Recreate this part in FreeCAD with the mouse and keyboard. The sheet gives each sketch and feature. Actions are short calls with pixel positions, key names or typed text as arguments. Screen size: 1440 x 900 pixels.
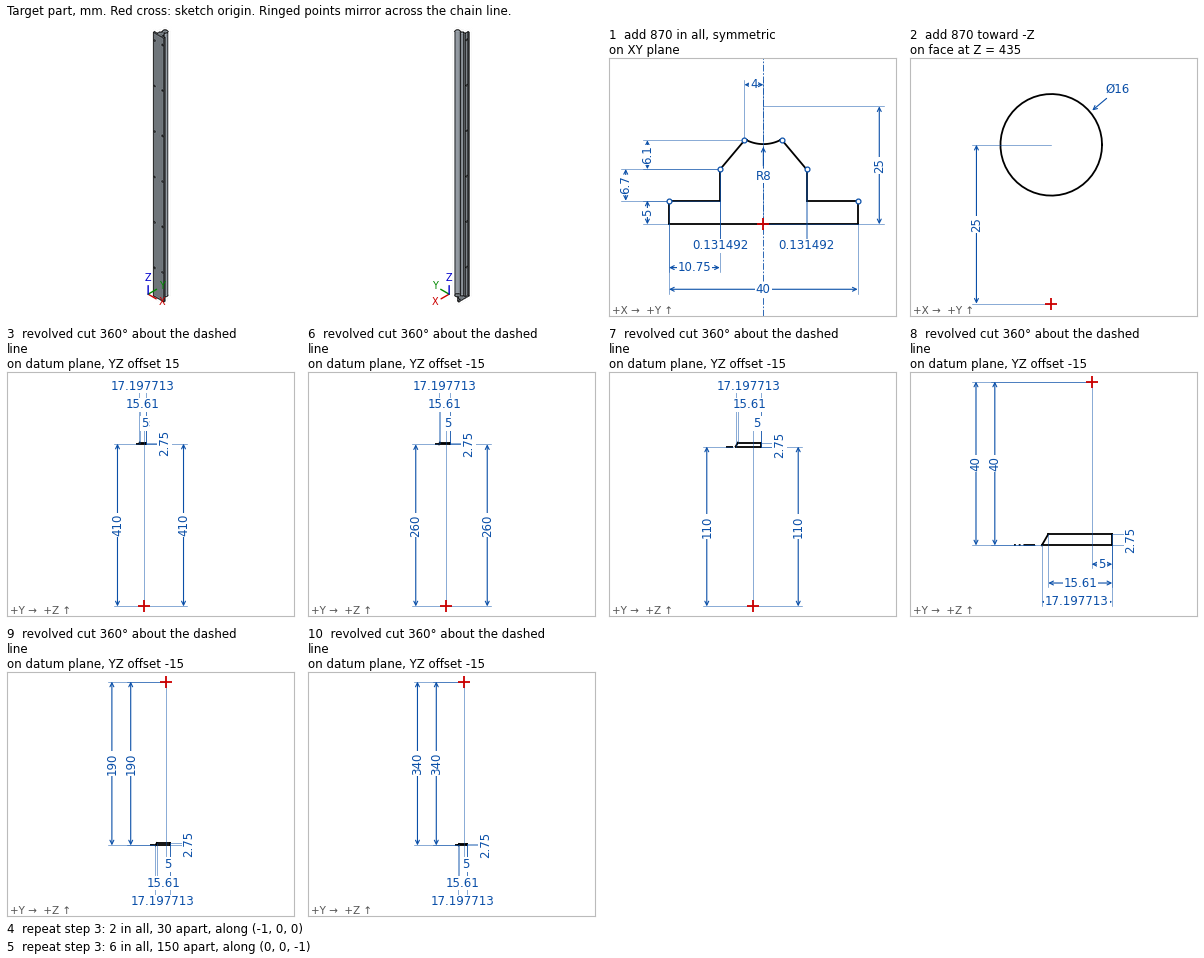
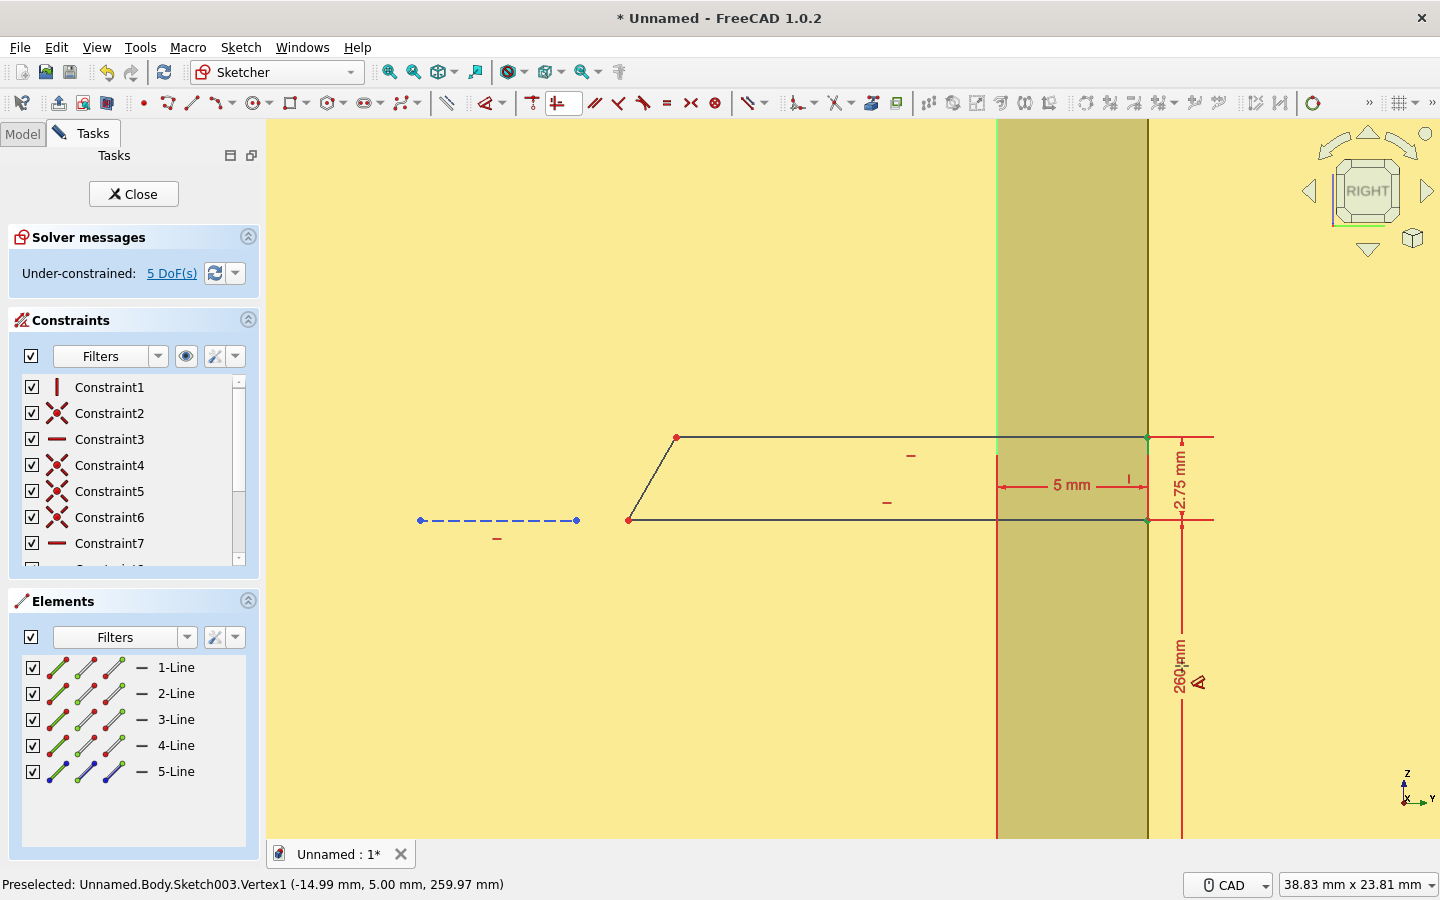
click(576, 521)
click(1031, 666)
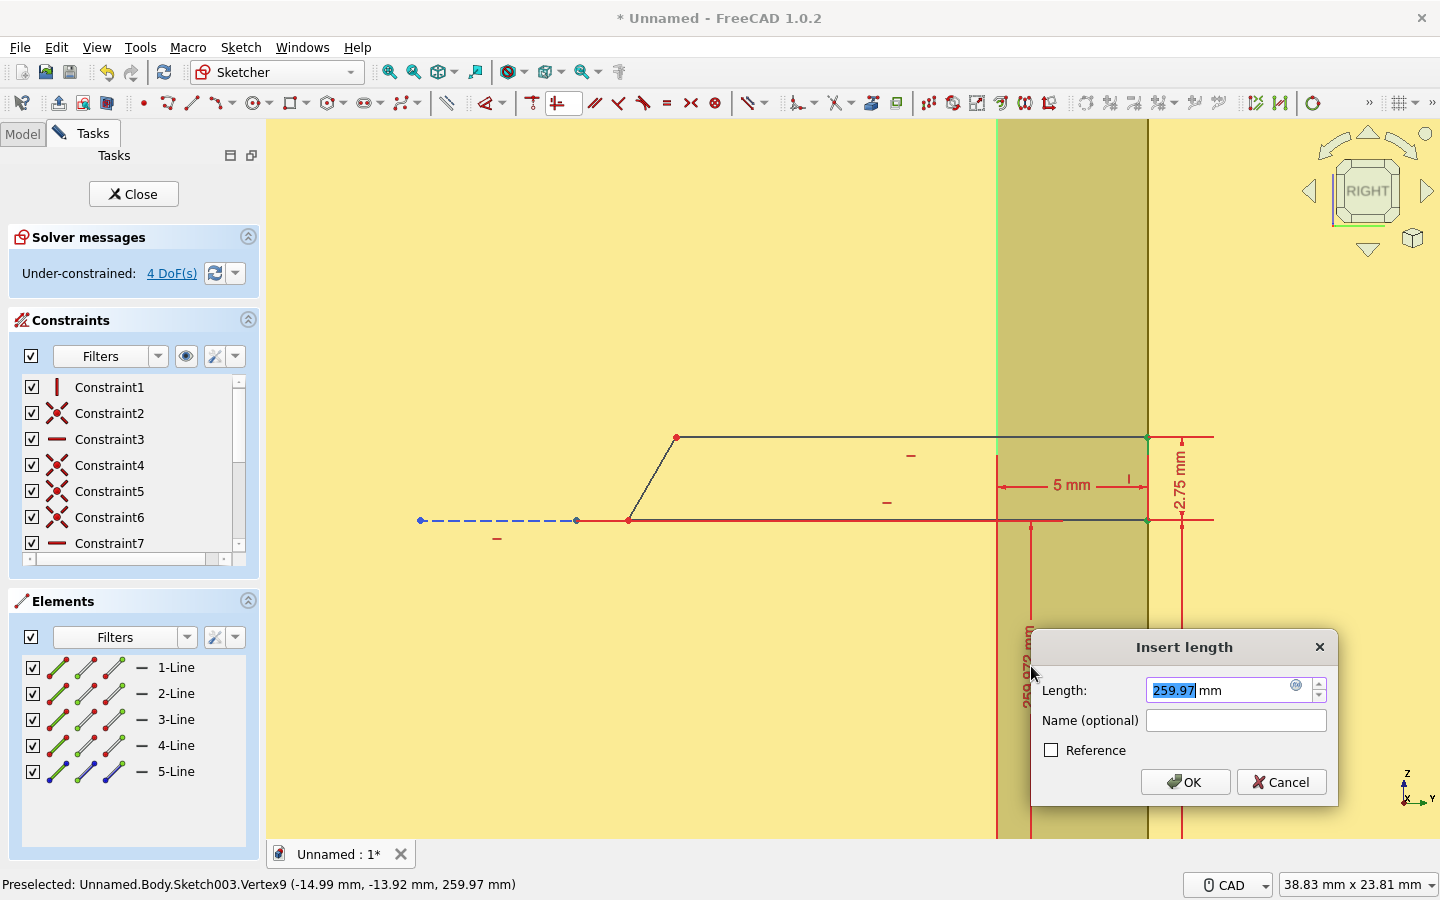
text(260)
key(Return)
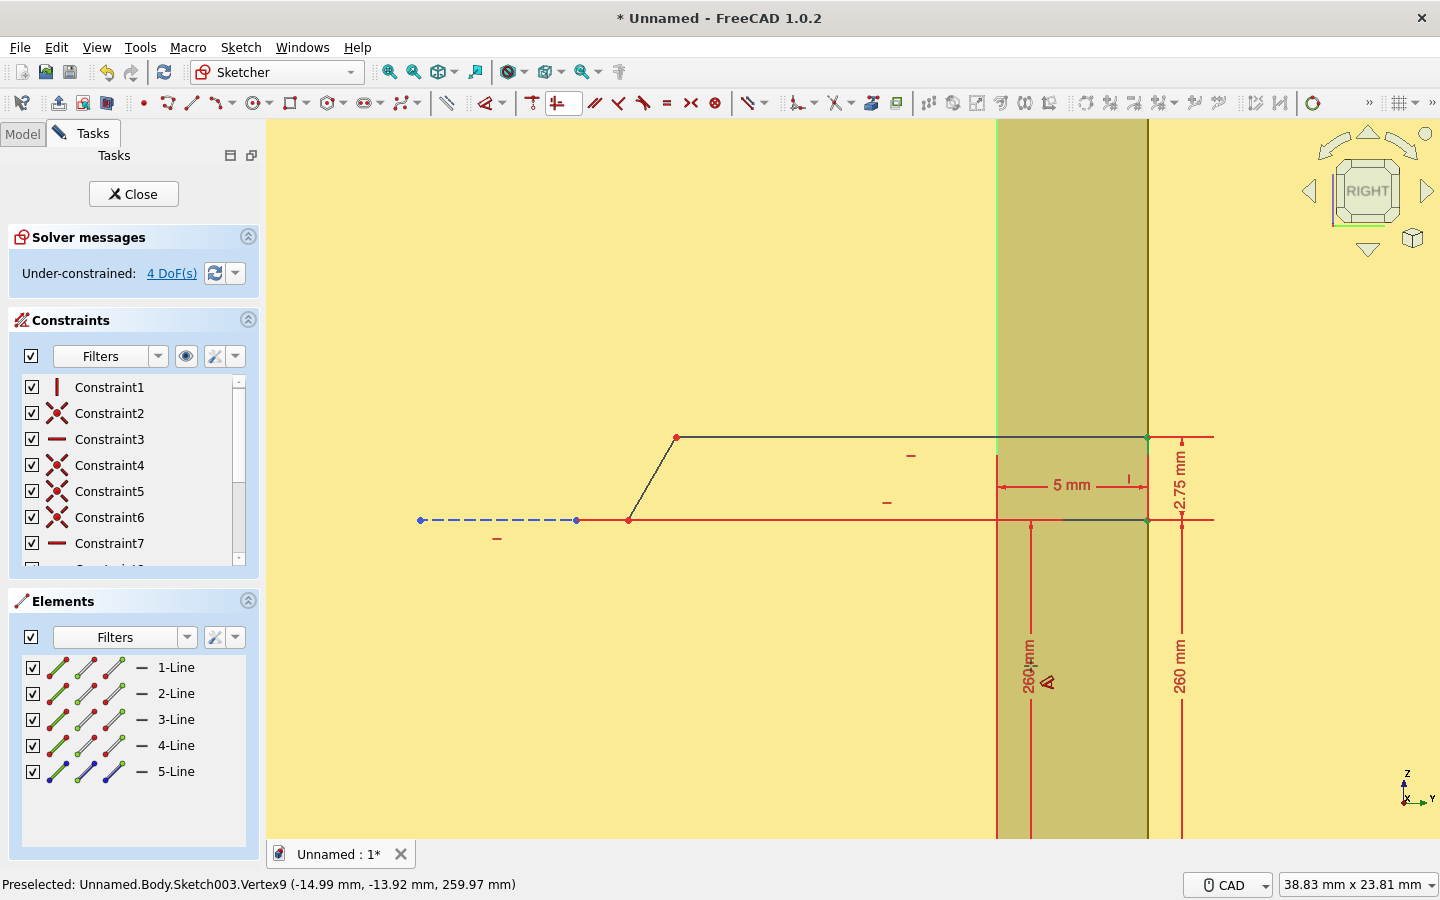
scroll(1006, 437, up, 2)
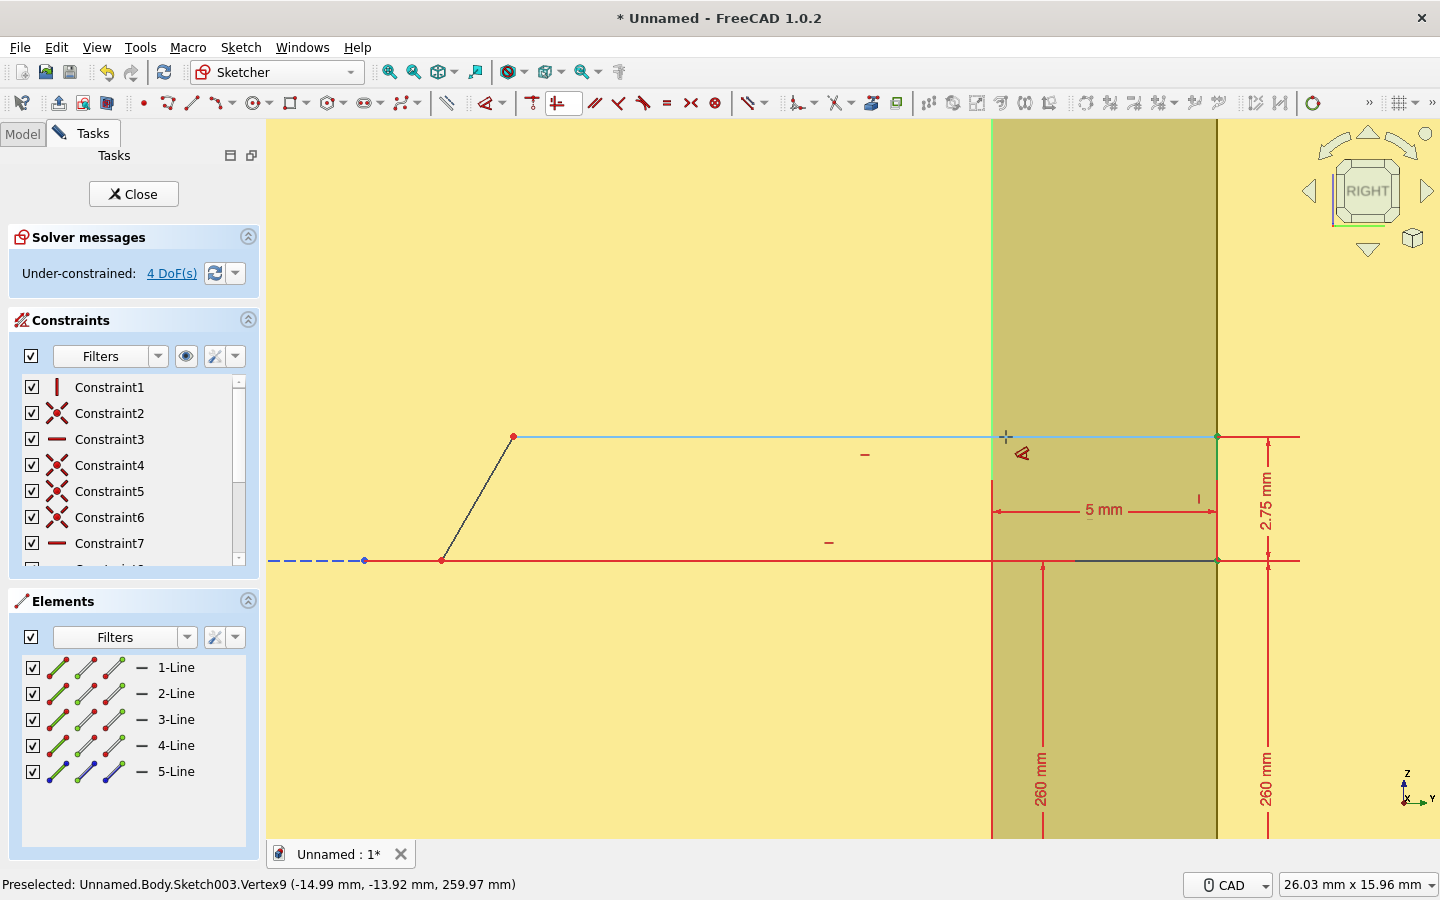
click(1006, 437)
click(865, 403)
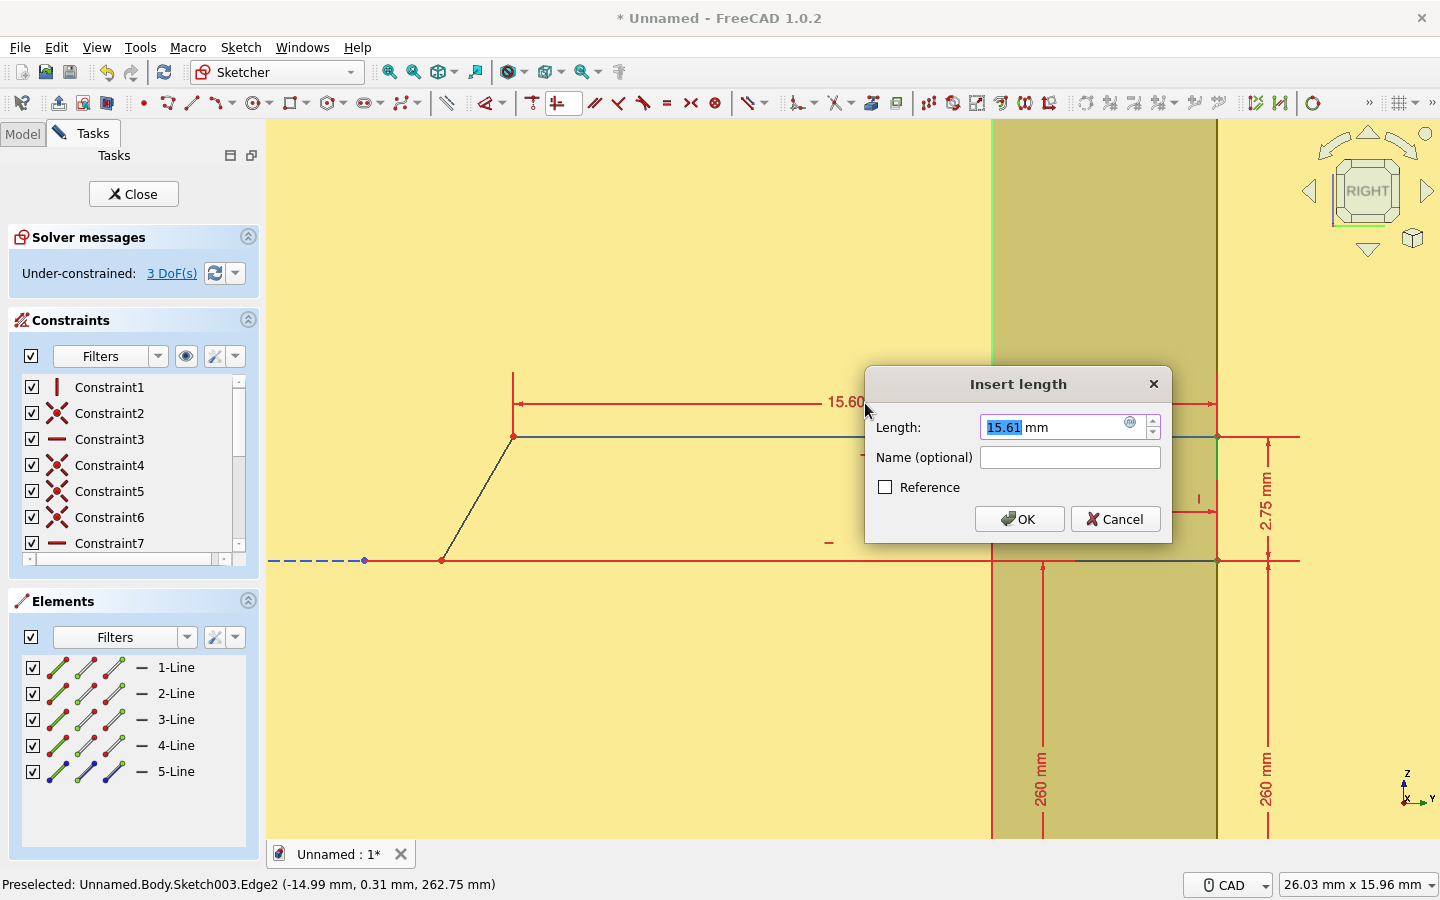
text(15.61)
key(Return)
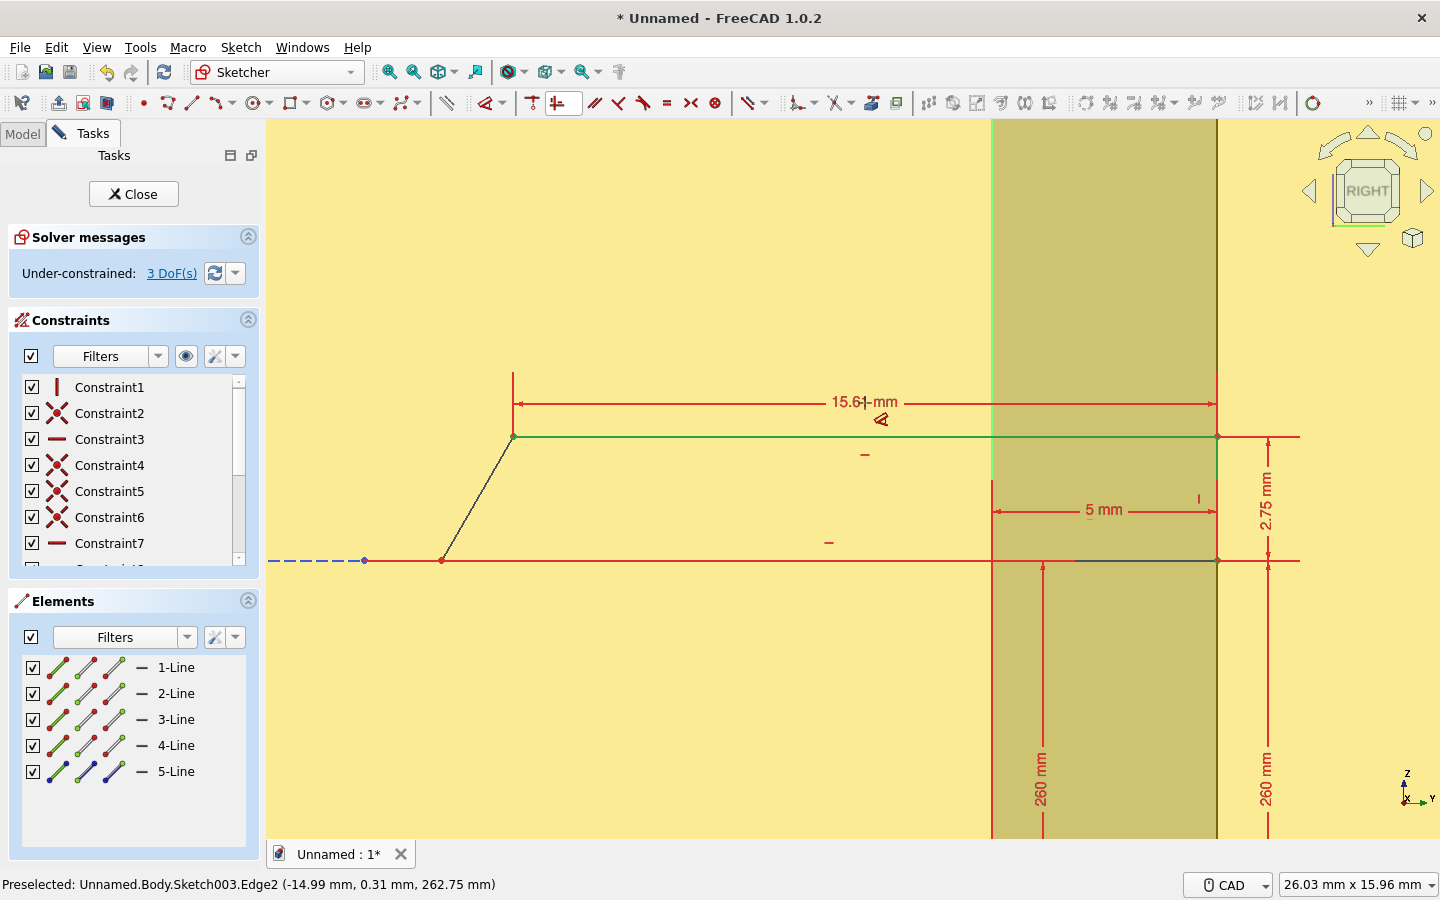
click(674, 561)
click(830, 595)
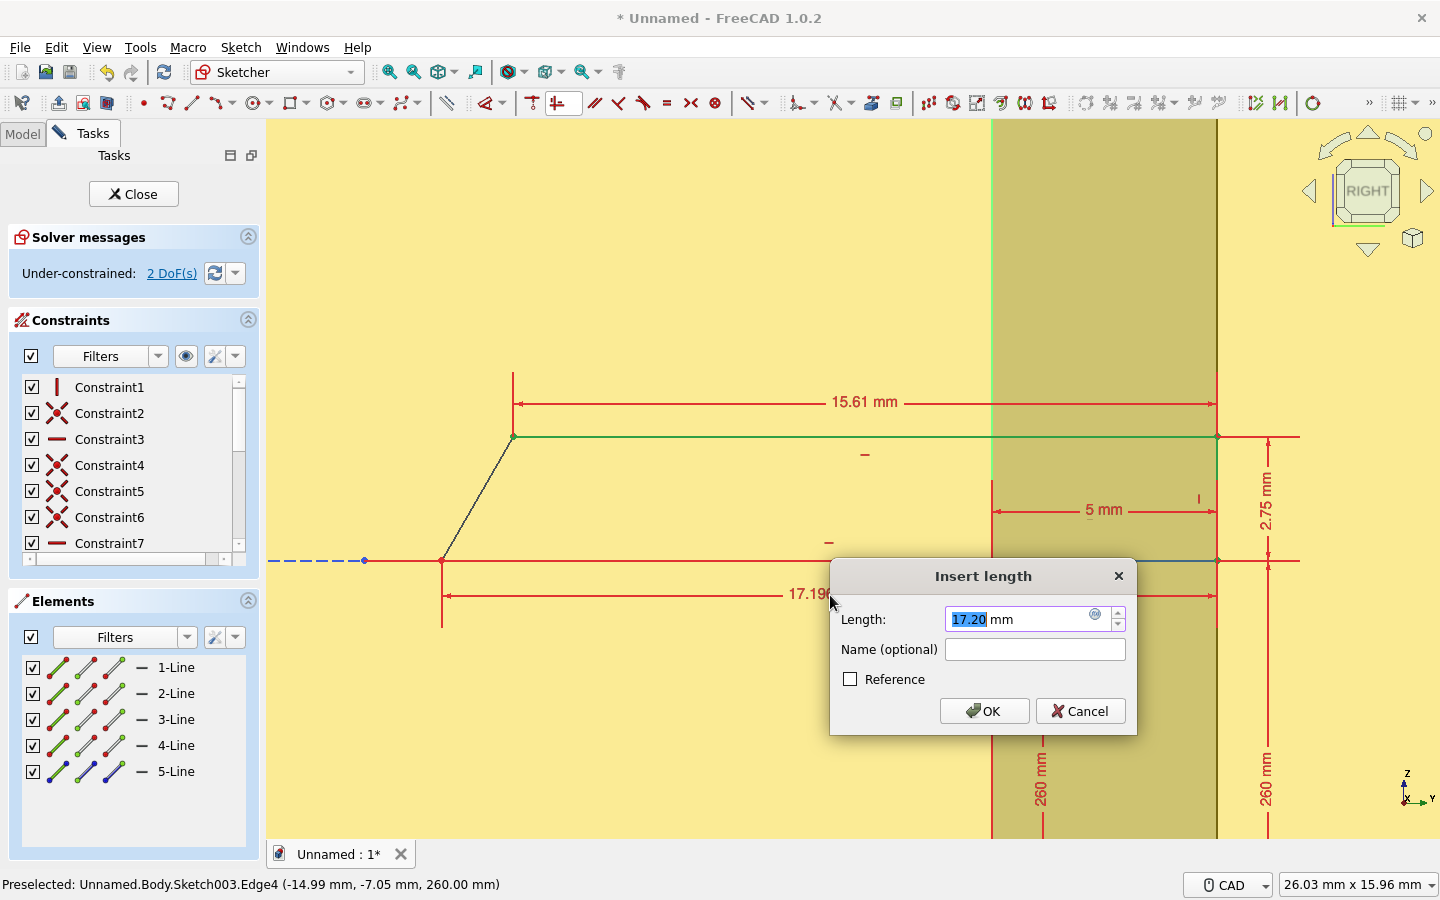
text(17.197713)
key(Return)
key(Escape)